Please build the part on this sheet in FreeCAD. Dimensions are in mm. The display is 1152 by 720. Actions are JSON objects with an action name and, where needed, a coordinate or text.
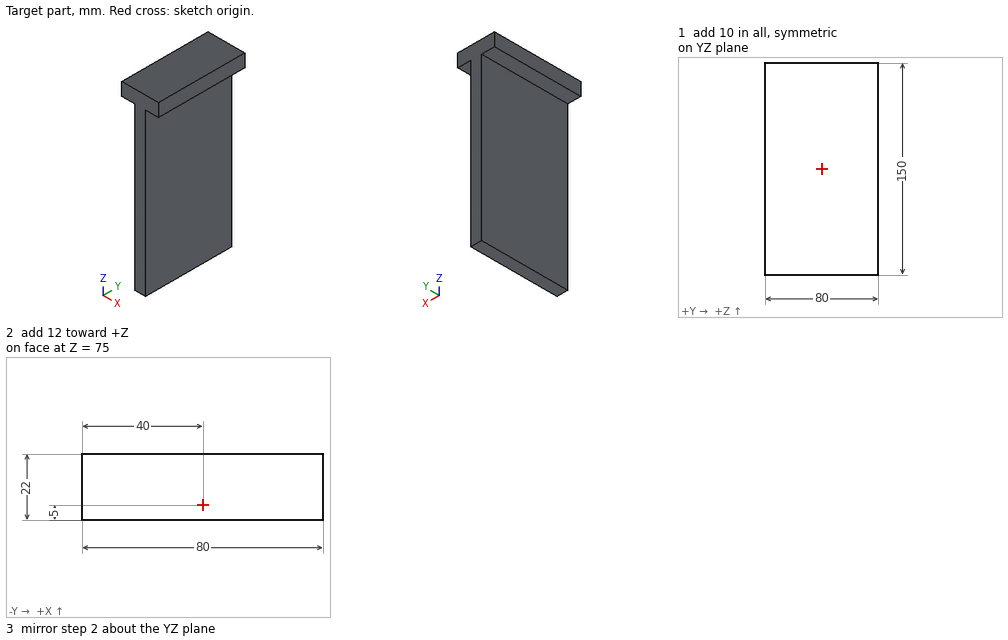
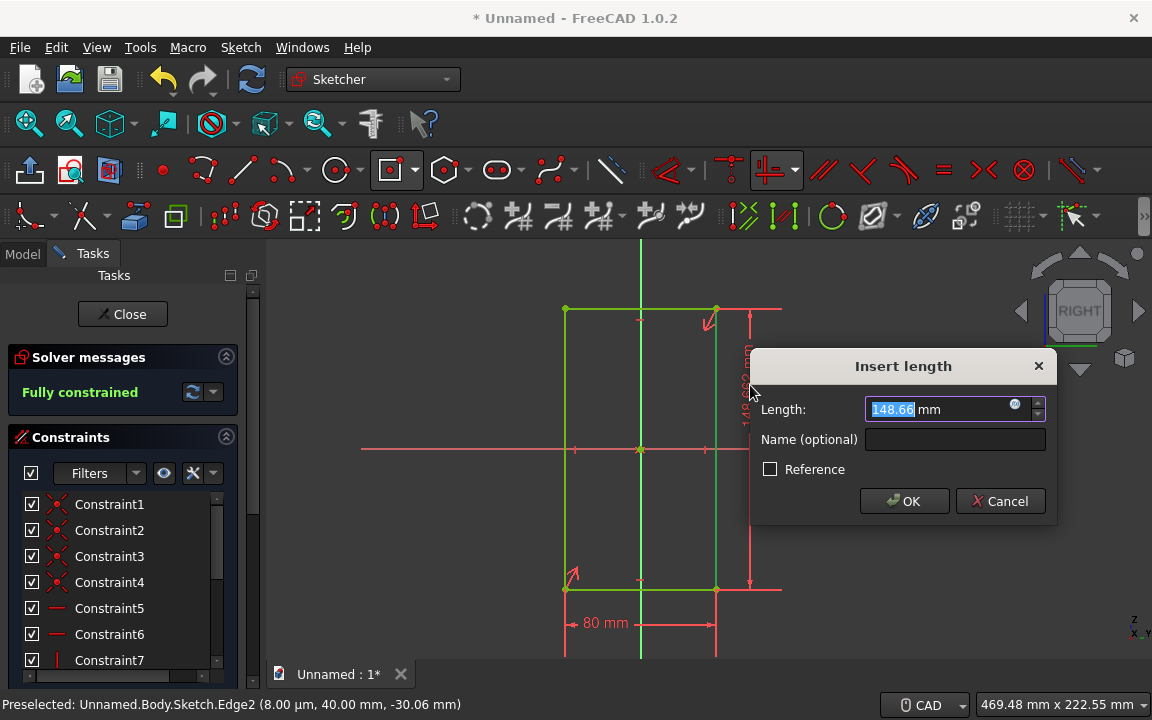
{"action": "type", "text": "150"}
{"action": "key", "text": "Return"}
{"action": "key", "text": "Escape"}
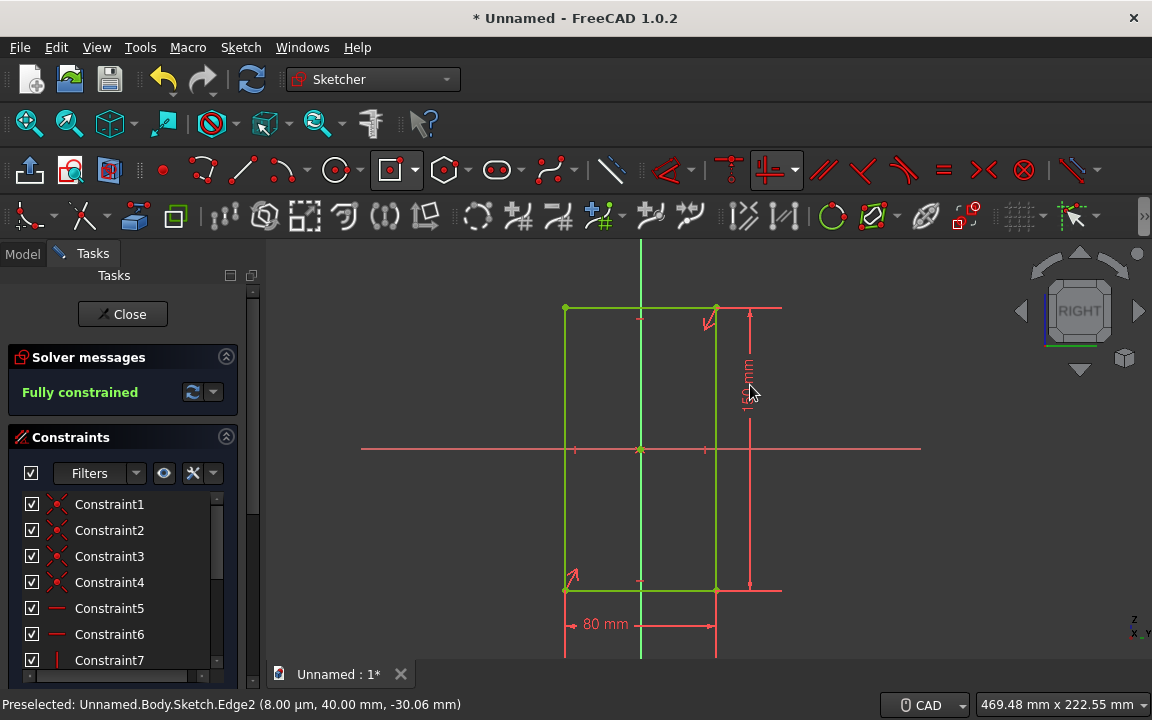
{"action": "left_click", "coordinate": [123, 314]}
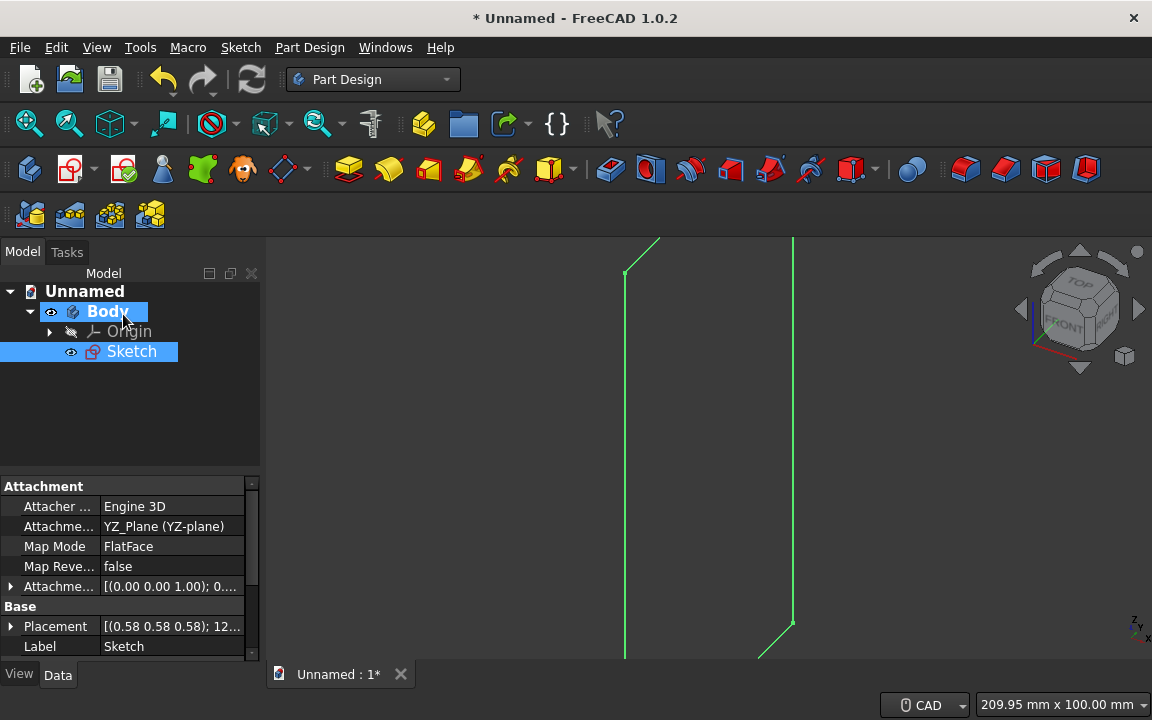
{"action": "left_click", "coordinate": [350, 170]}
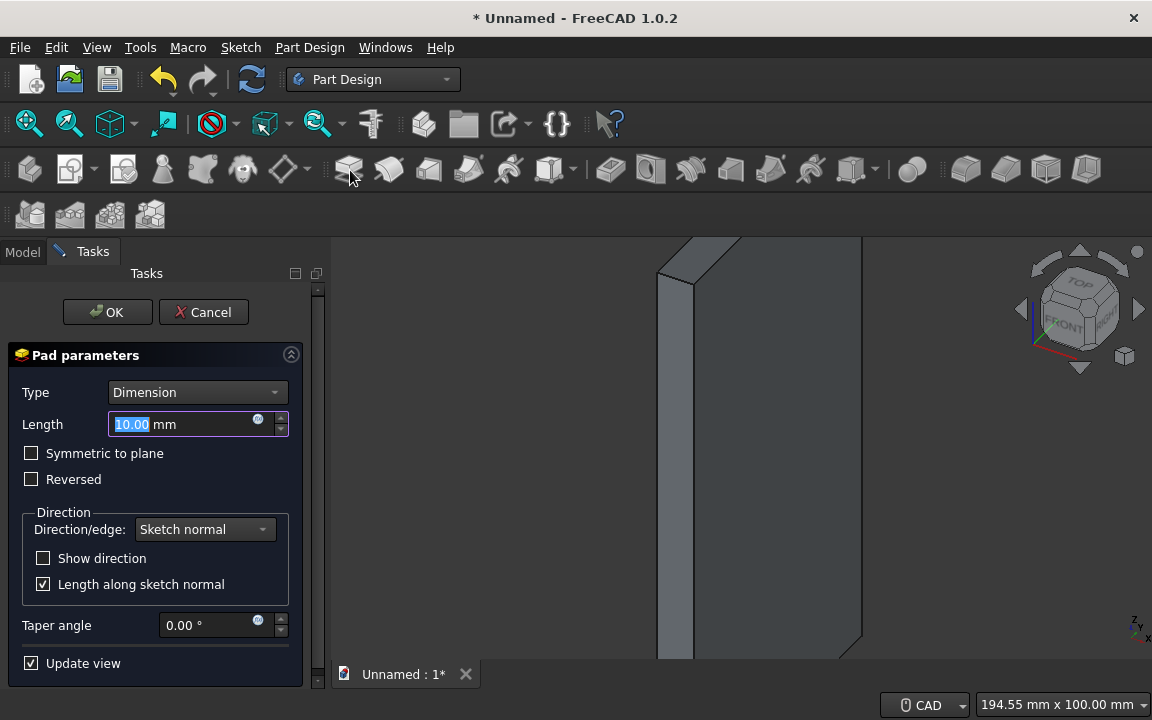
{"action": "type", "text": "10"}
{"action": "key", "text": "Tab"}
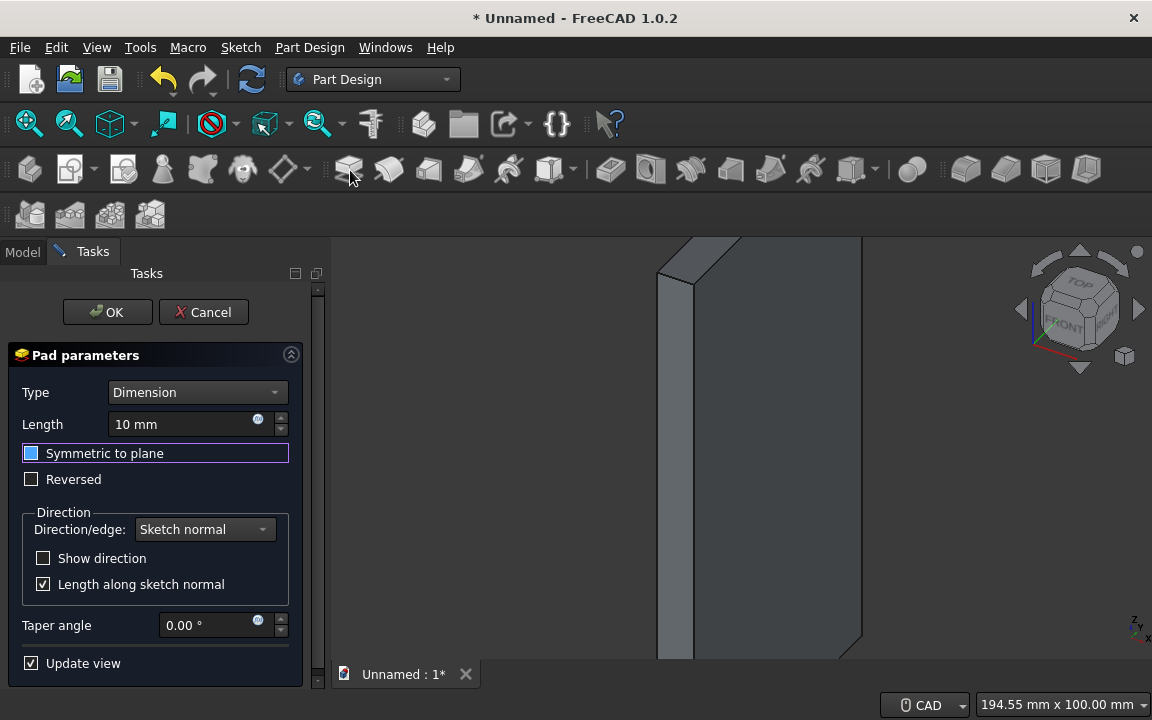
{"action": "left_click", "coordinate": [30, 453]}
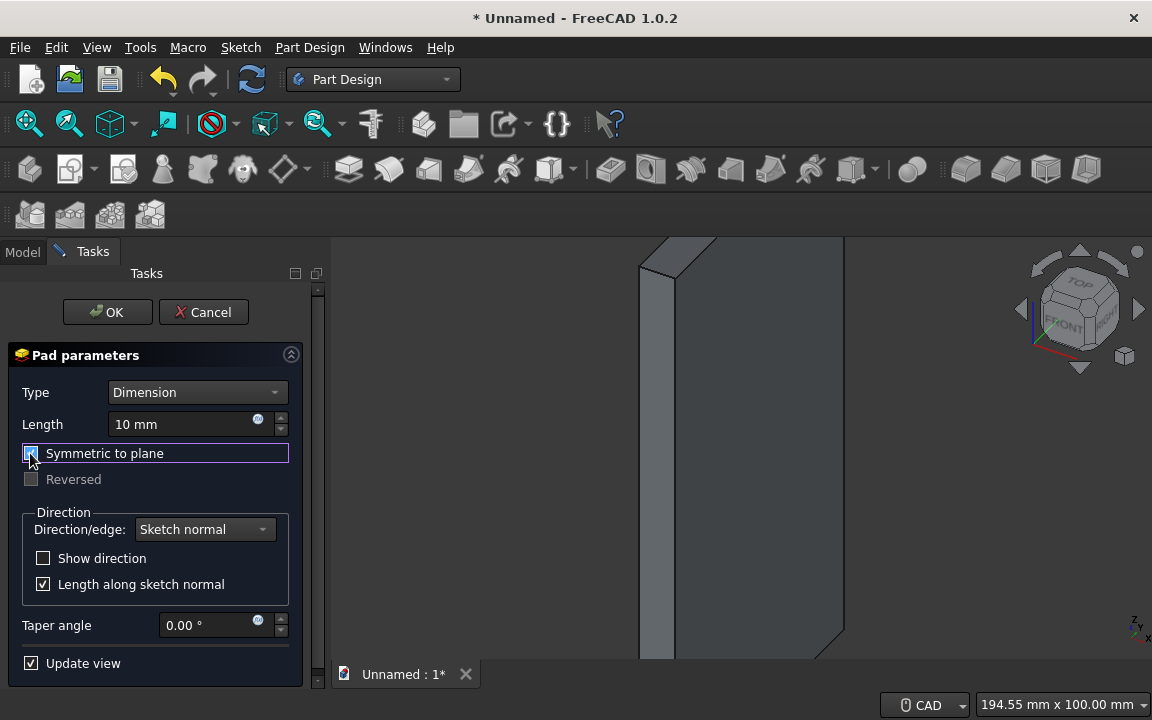
{"action": "left_click", "coordinate": [108, 312]}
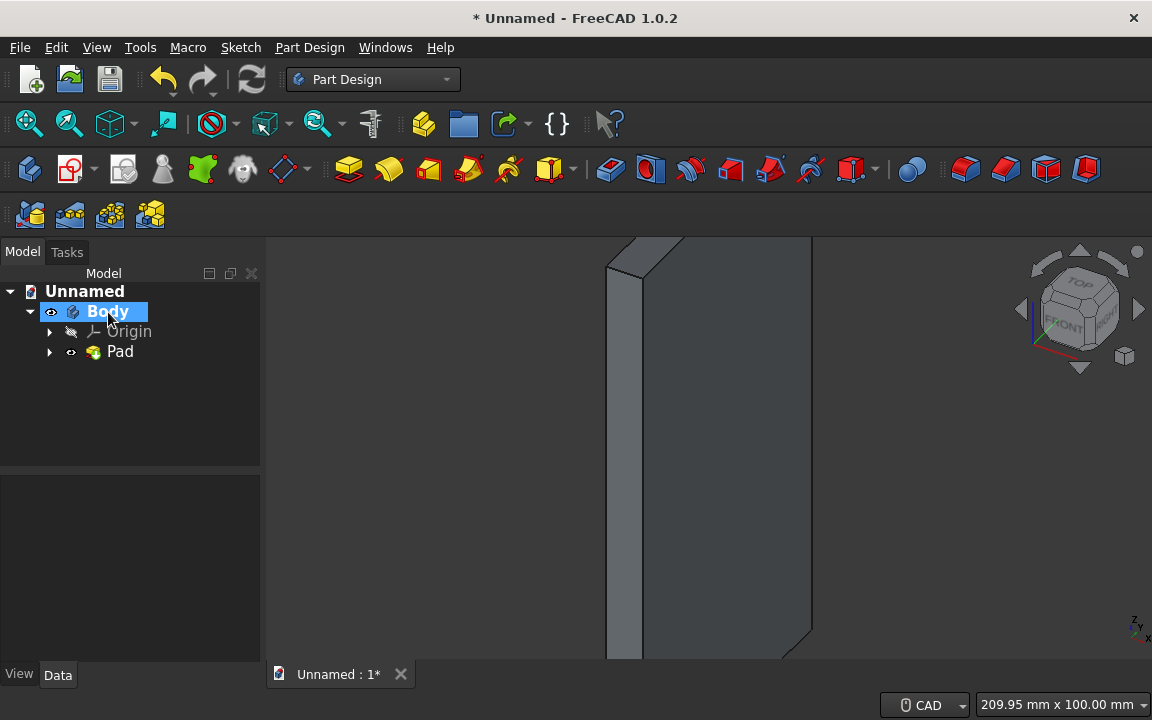
{"action": "left_click", "coordinate": [30, 124]}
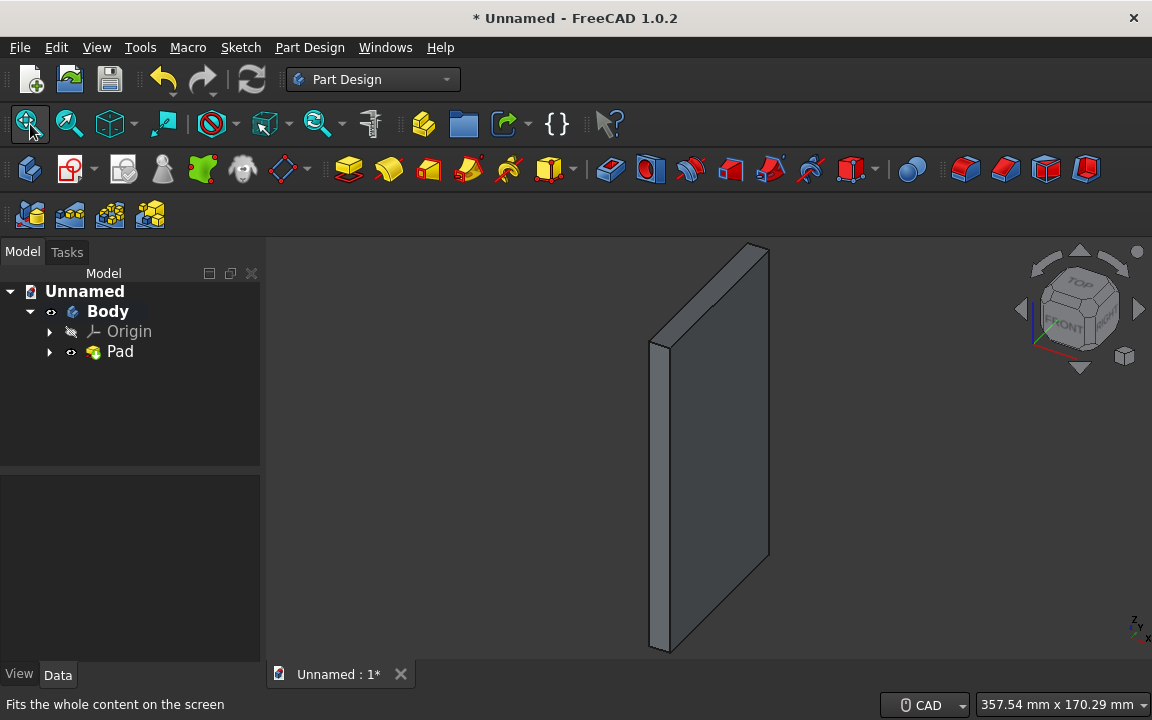
{"action": "left_click", "coordinate": [737, 267]}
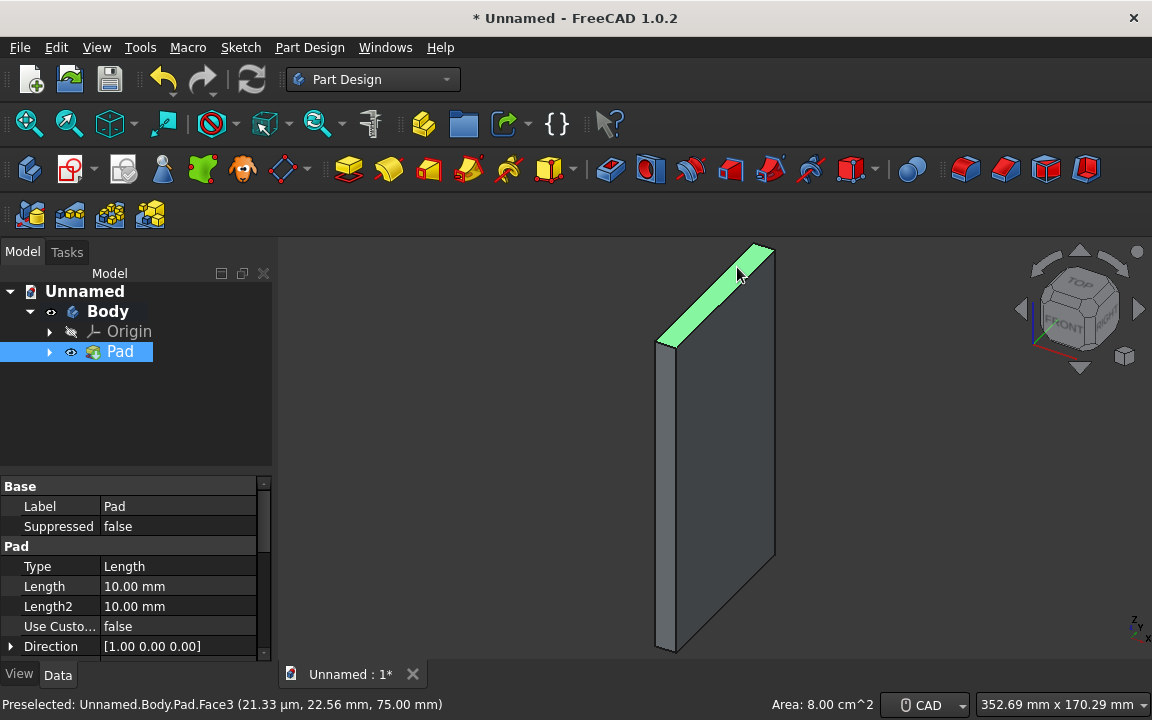
{"action": "left_click", "coordinate": [70, 170]}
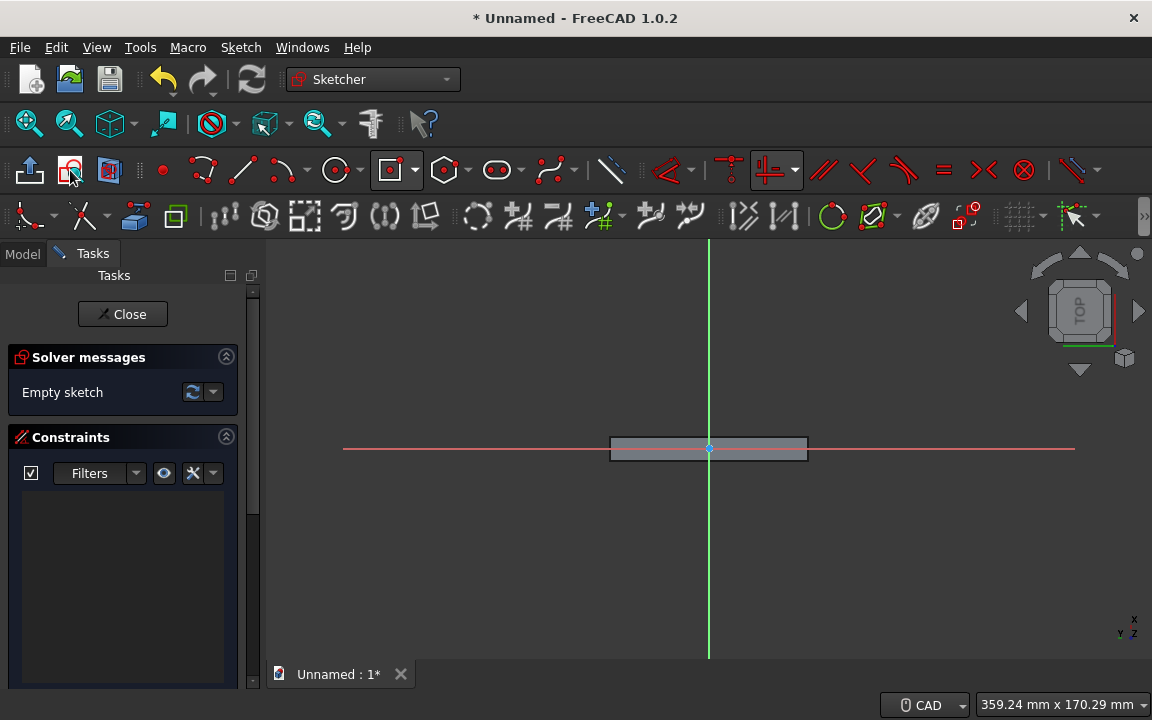
{"action": "scroll", "coordinate": [749, 426], "scroll_direction": "up", "scroll_amount": 5}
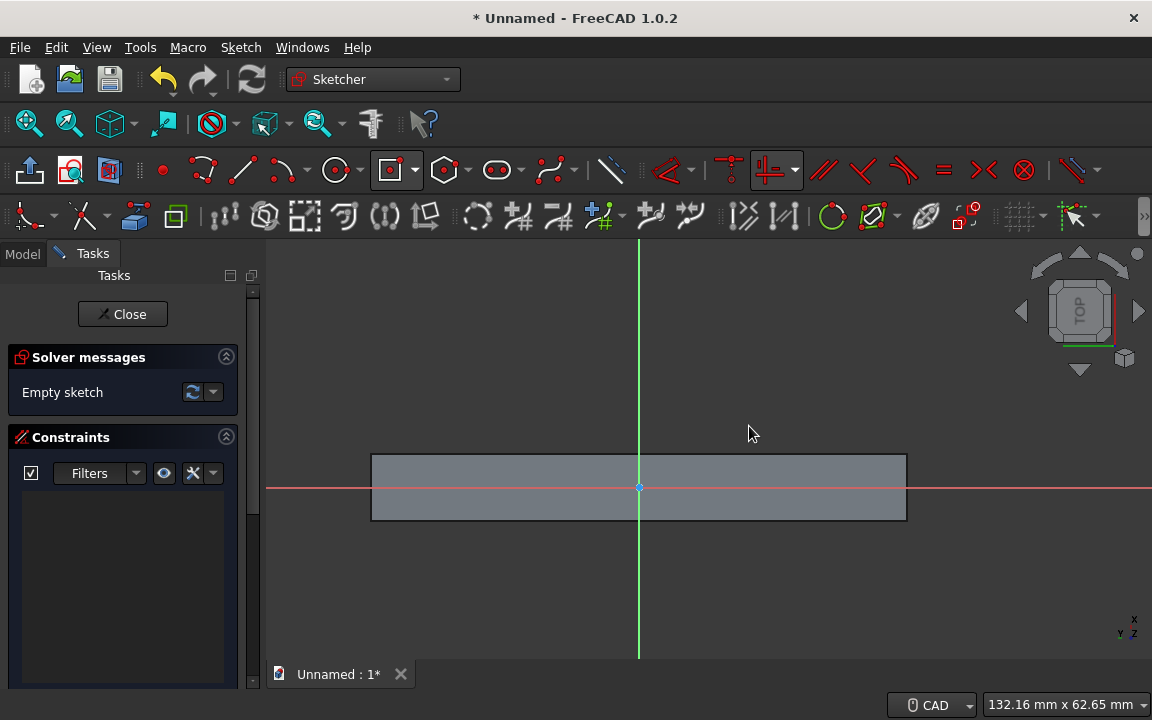
{"action": "left_click", "coordinate": [418, 170]}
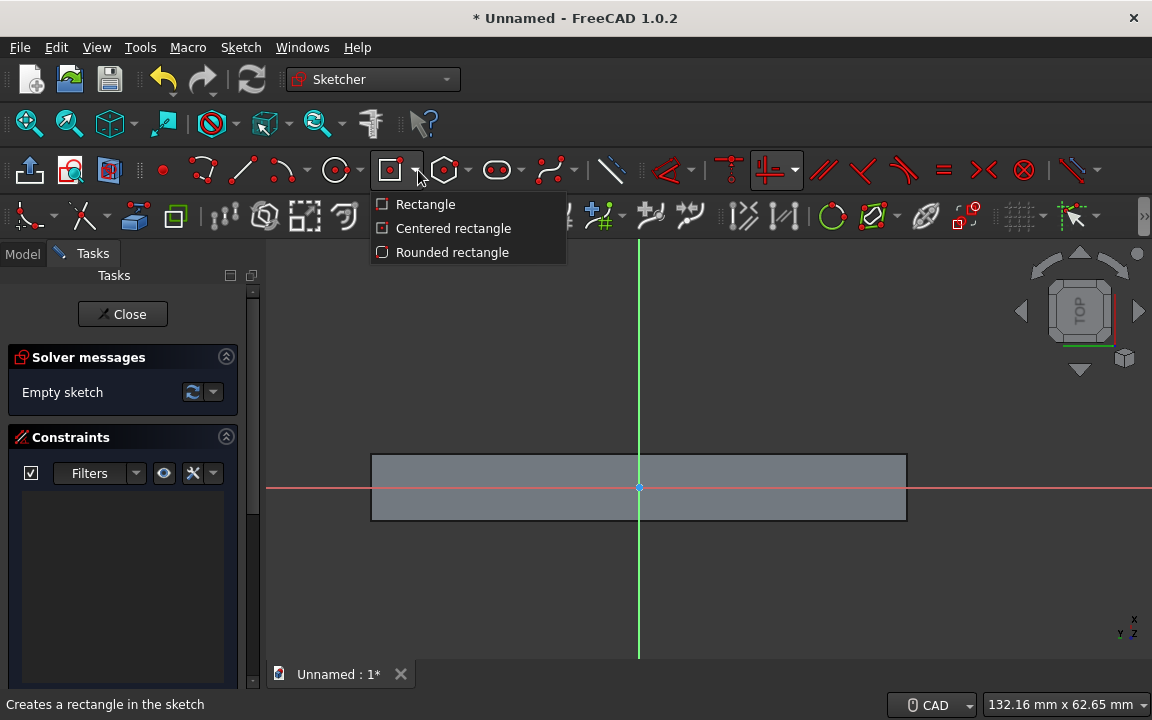
{"action": "left_click", "coordinate": [468, 204]}